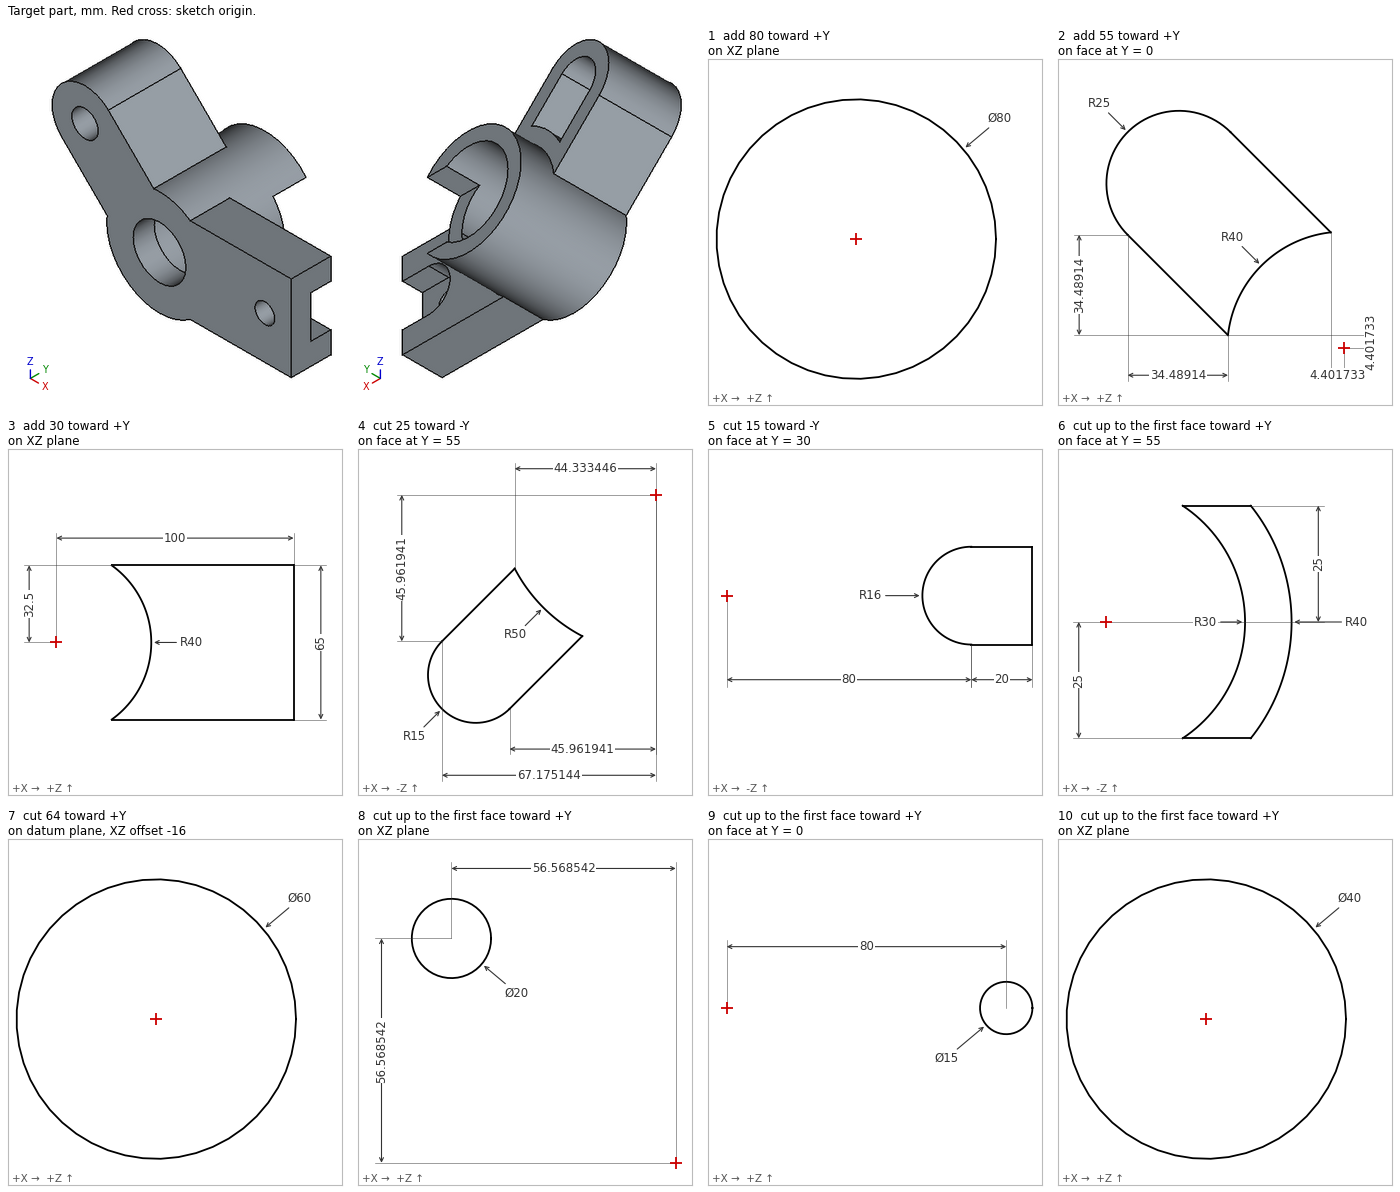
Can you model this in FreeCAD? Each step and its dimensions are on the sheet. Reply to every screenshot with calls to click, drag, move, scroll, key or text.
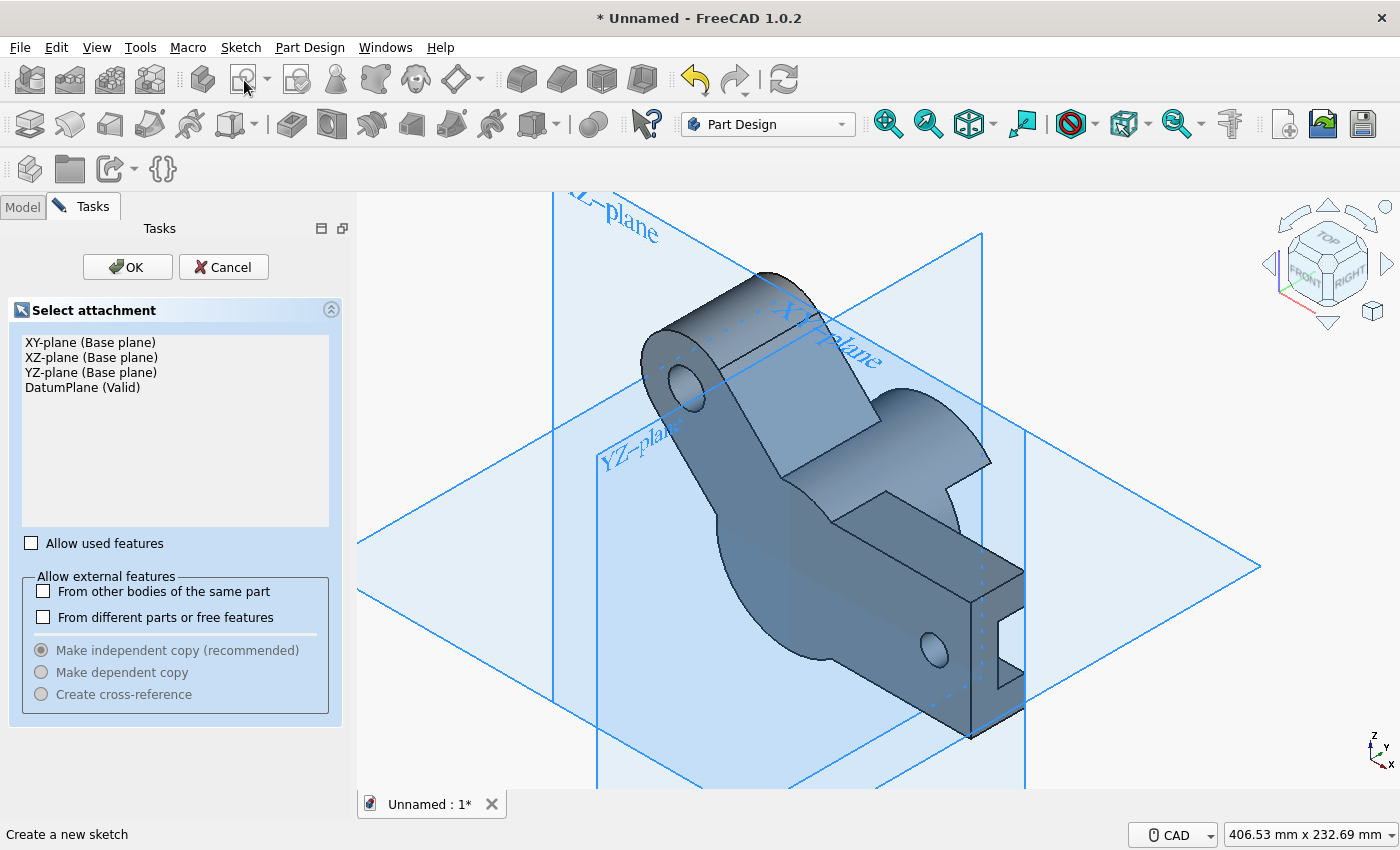
click(82, 358)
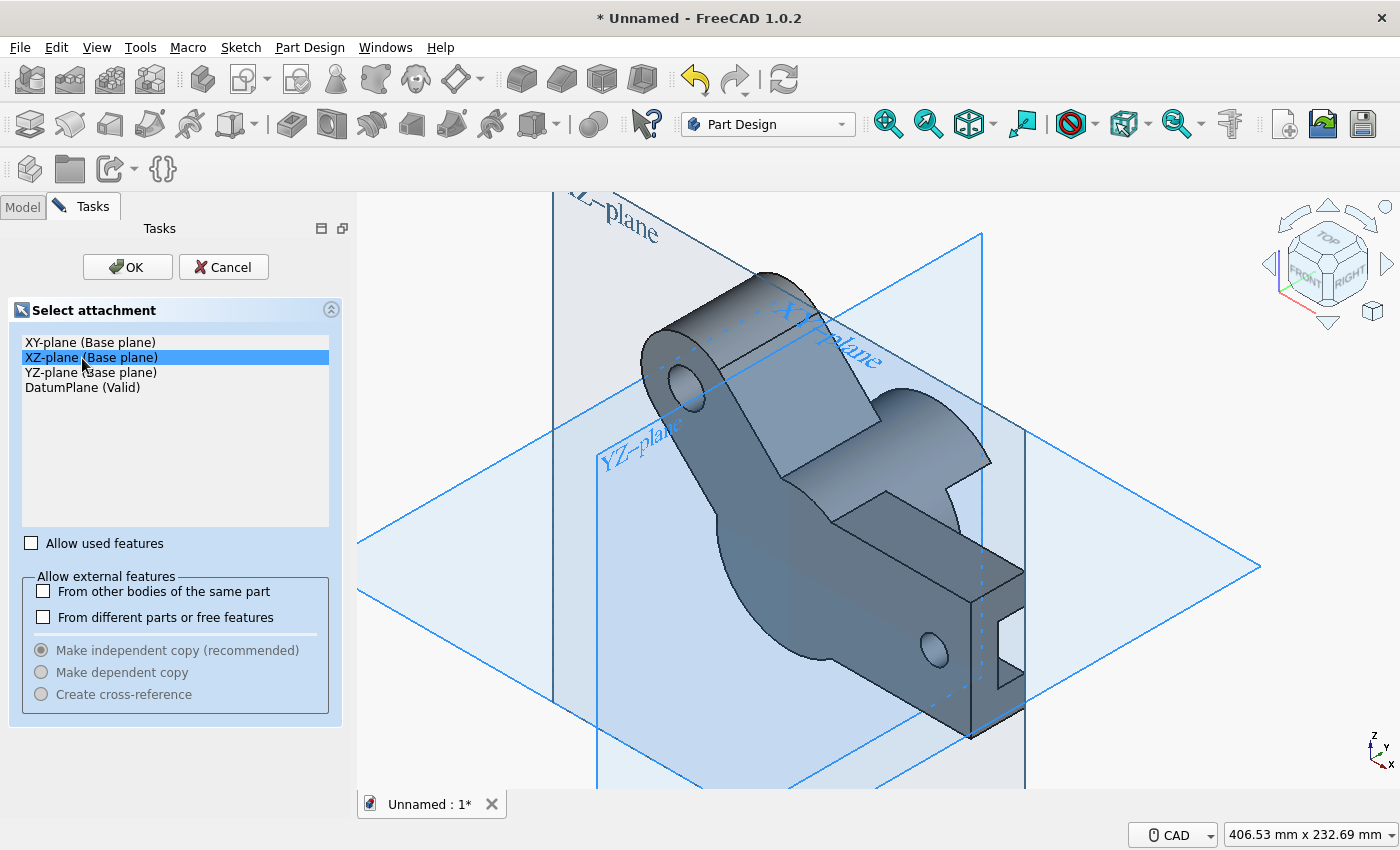
click(128, 267)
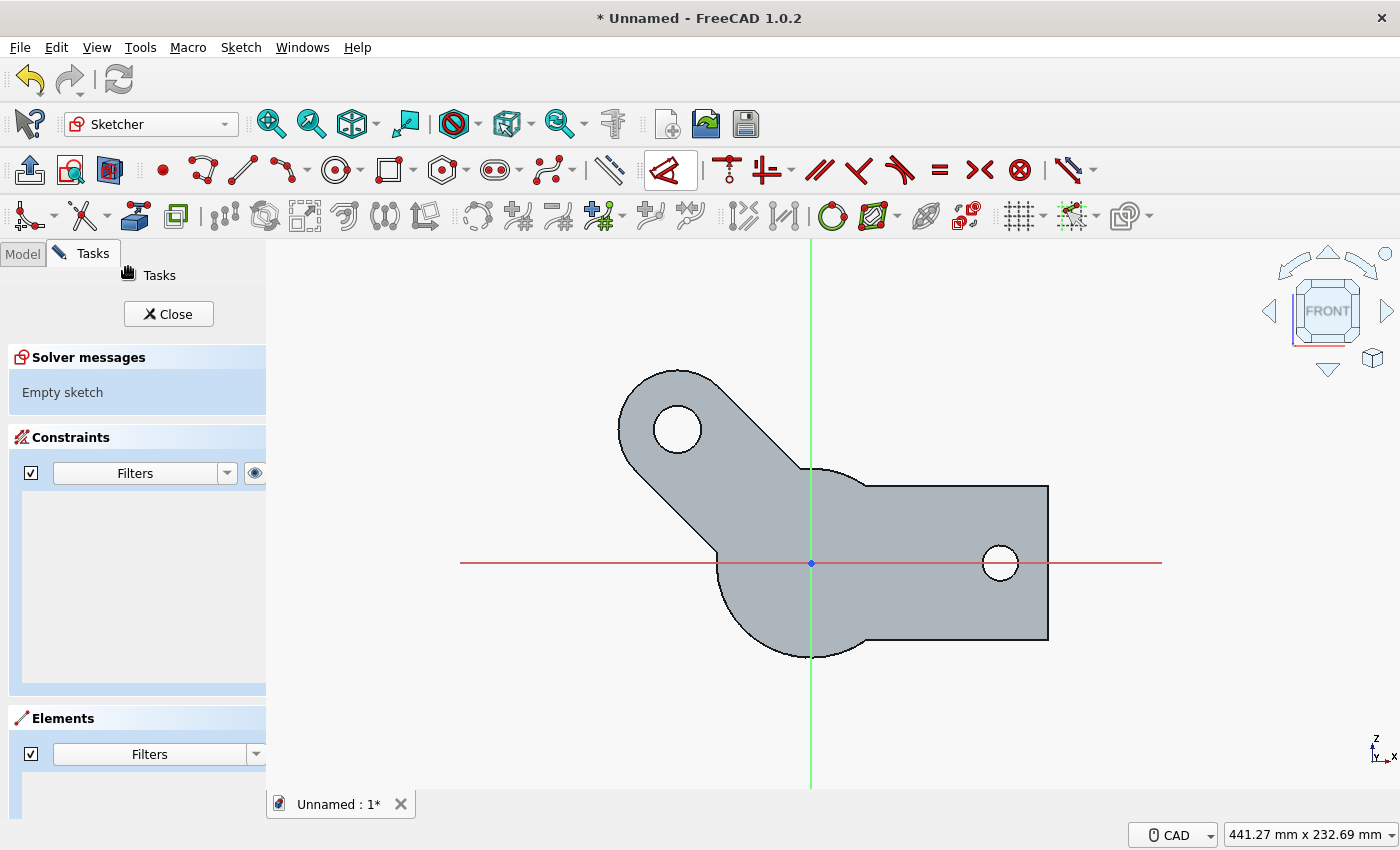
scroll(827, 579, up, 7)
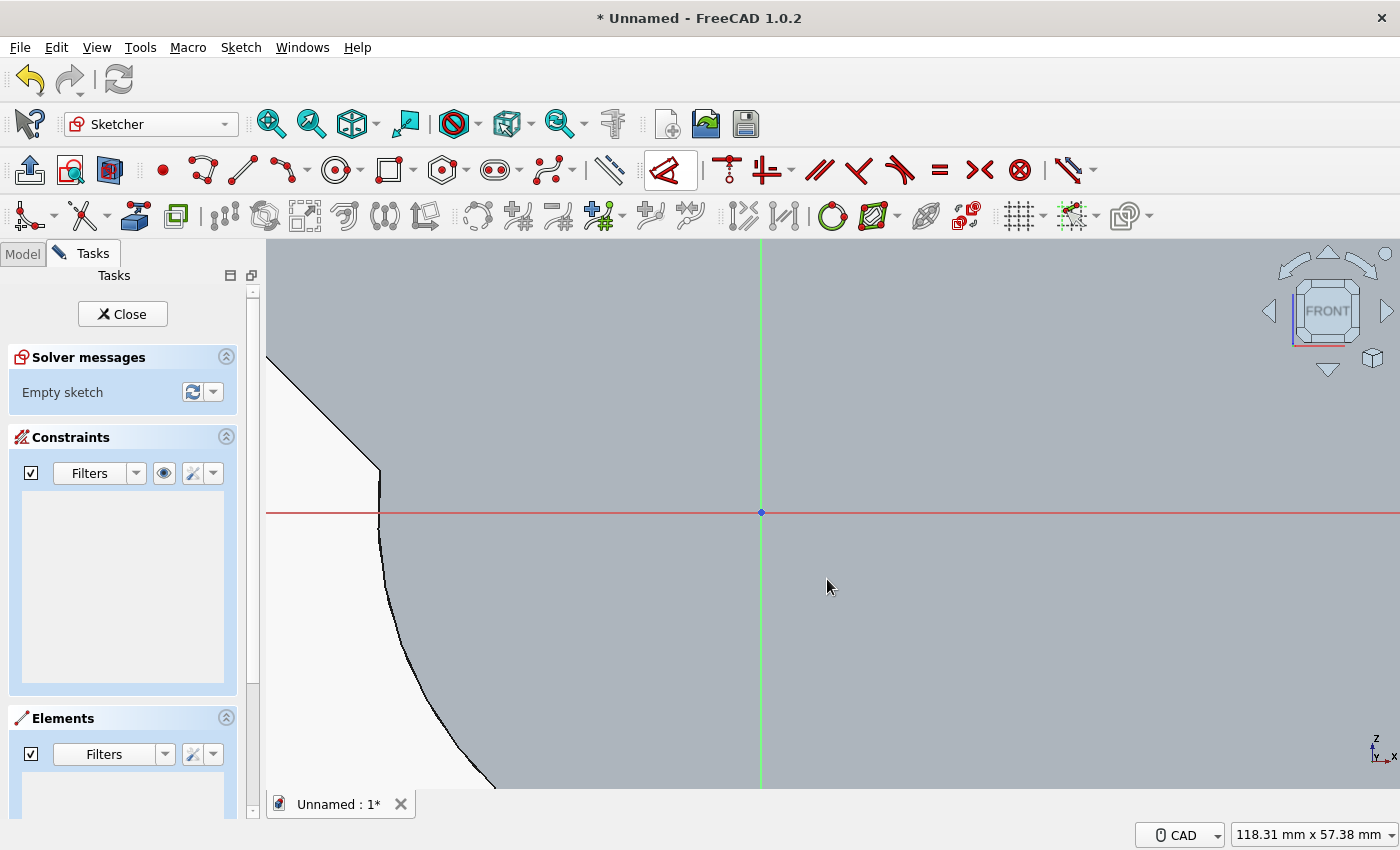
key(g)
key(c)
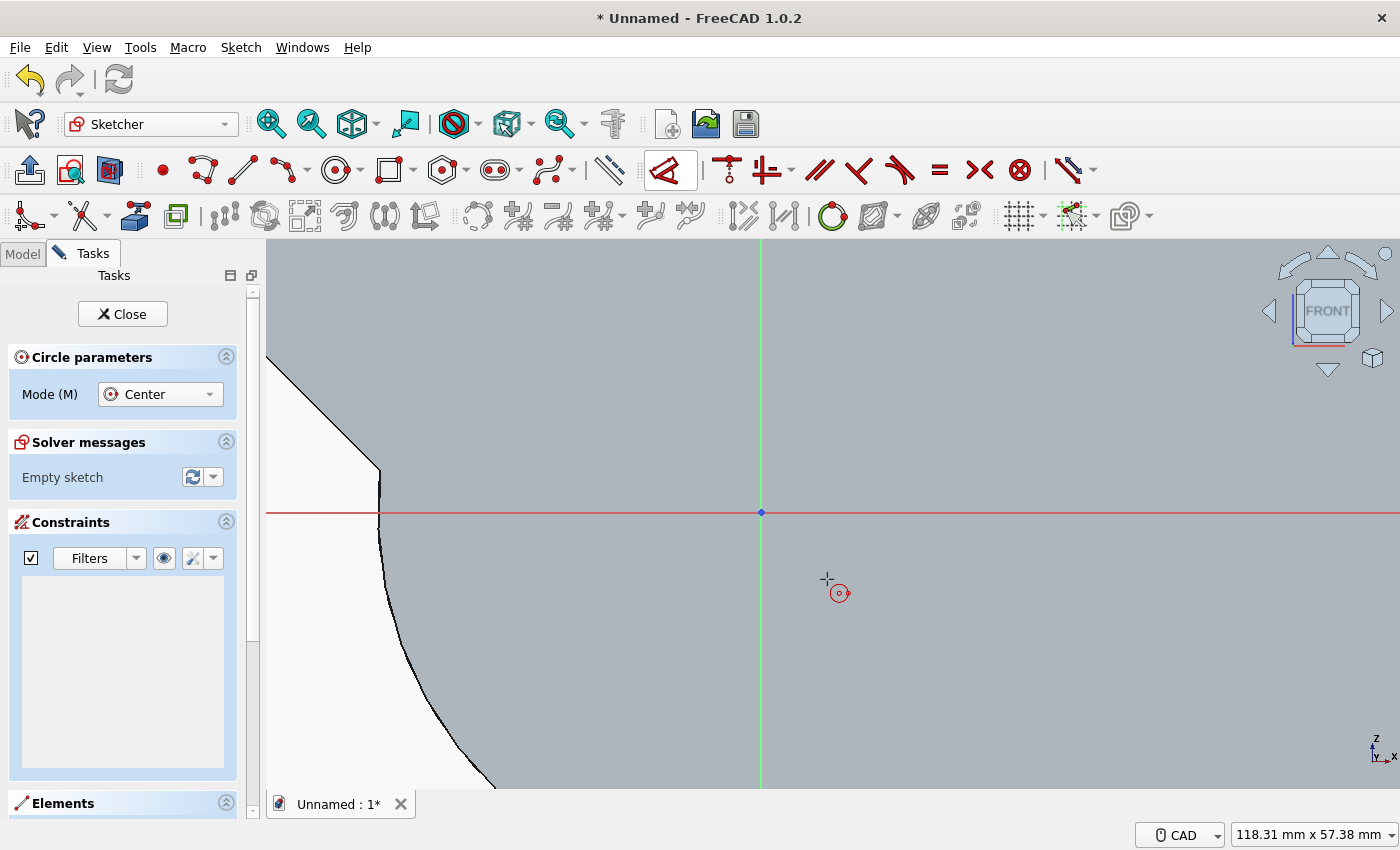
click(761, 513)
click(897, 377)
key(Escape)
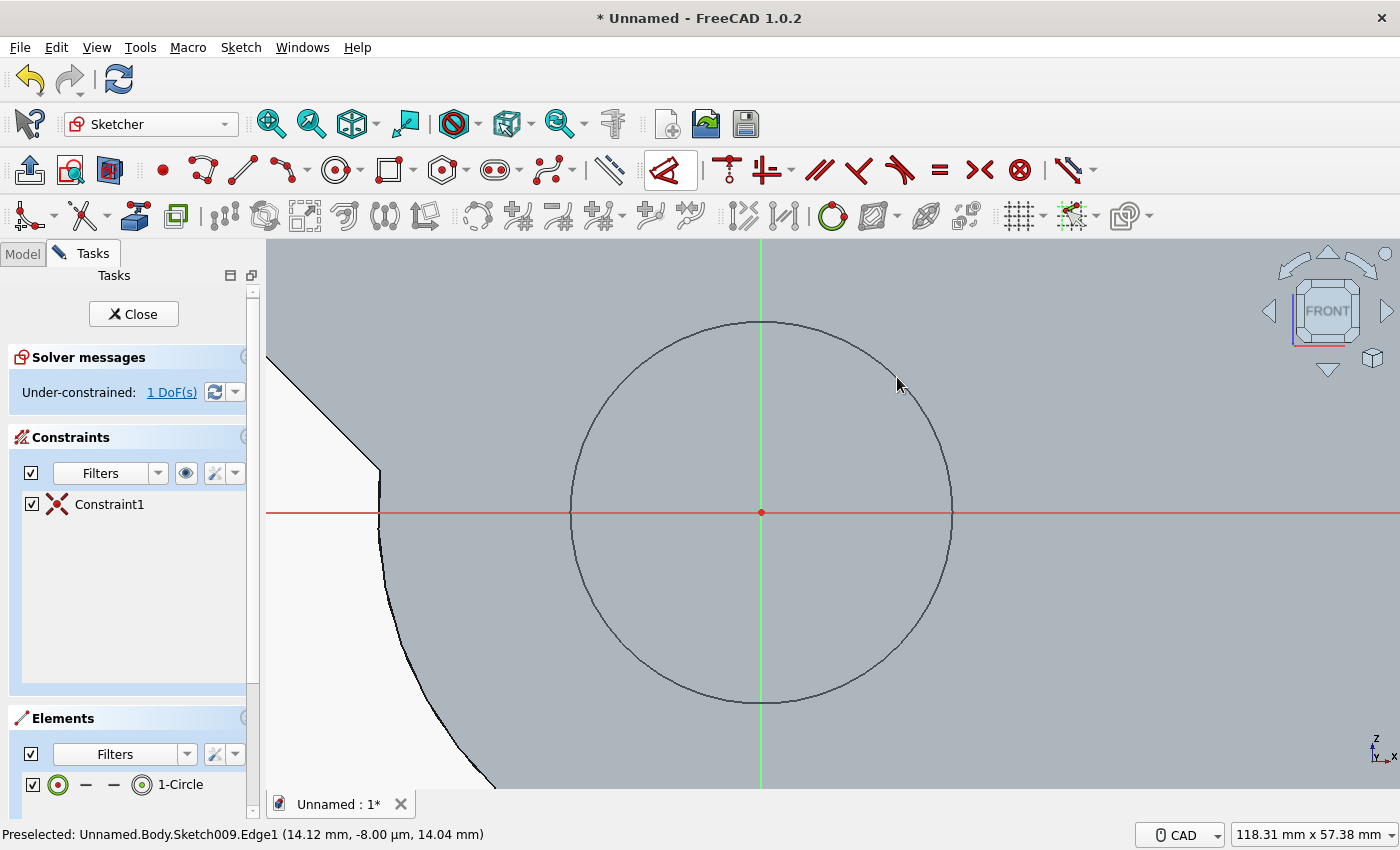
click(896, 377)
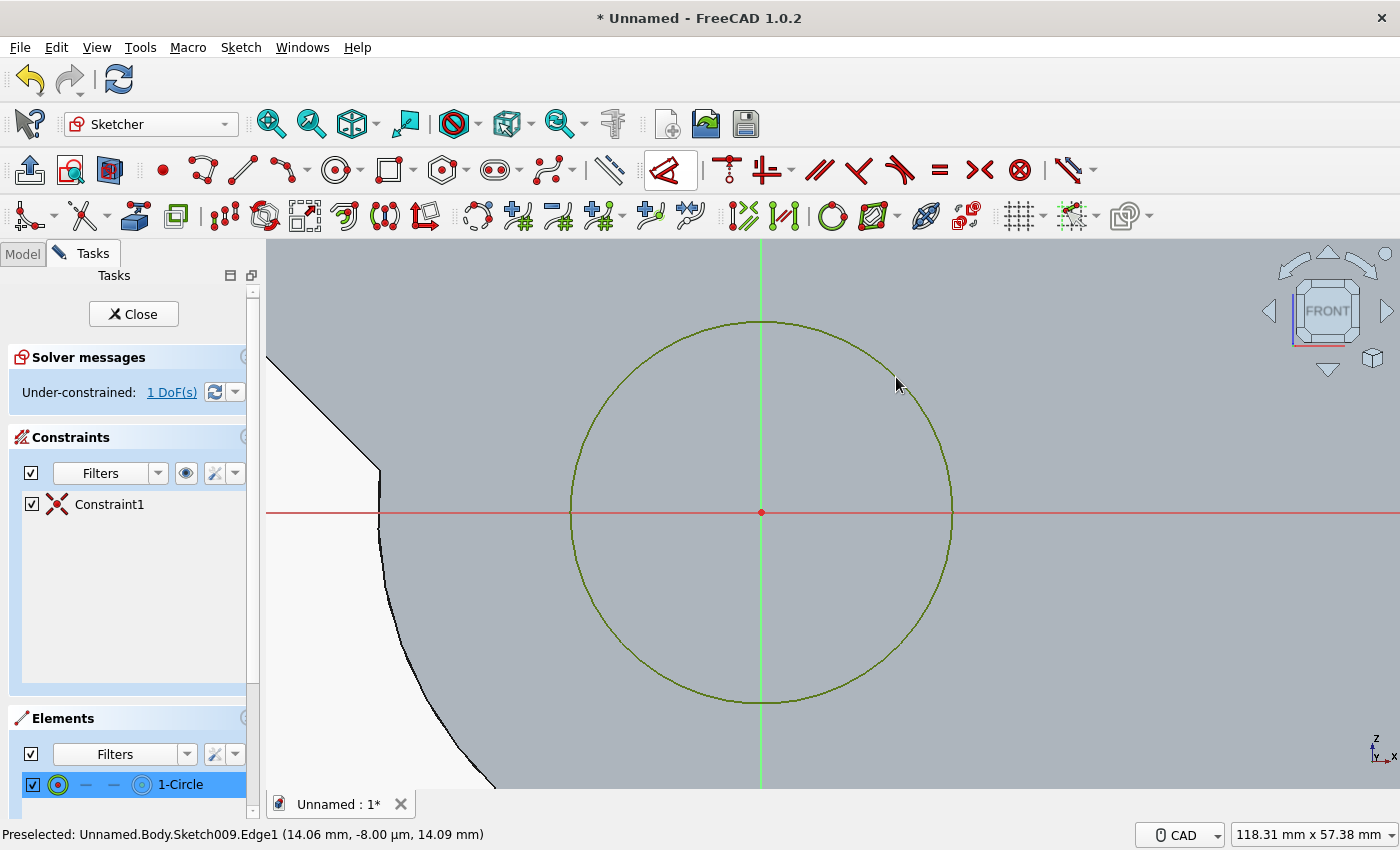
click(692, 170)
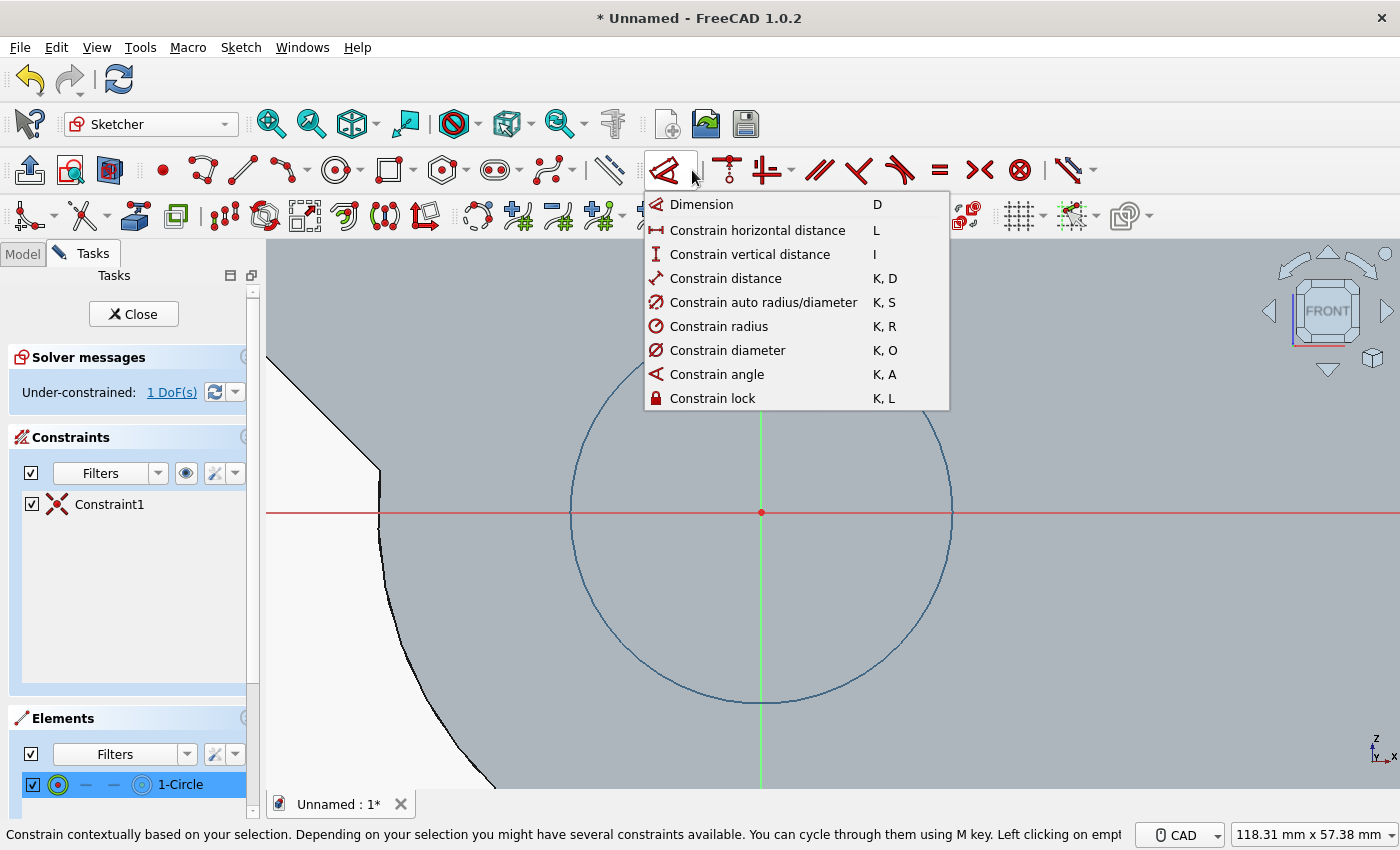
click(797, 350)